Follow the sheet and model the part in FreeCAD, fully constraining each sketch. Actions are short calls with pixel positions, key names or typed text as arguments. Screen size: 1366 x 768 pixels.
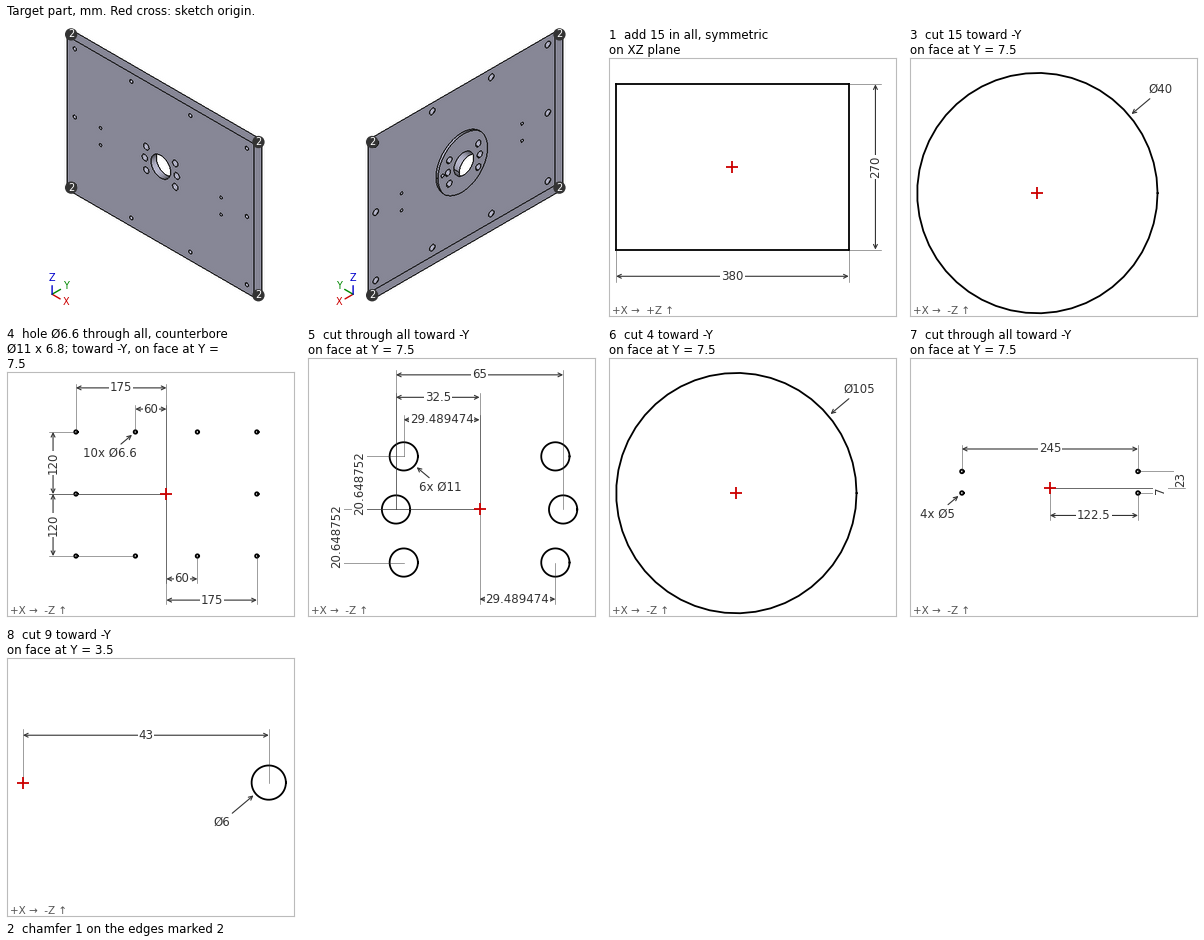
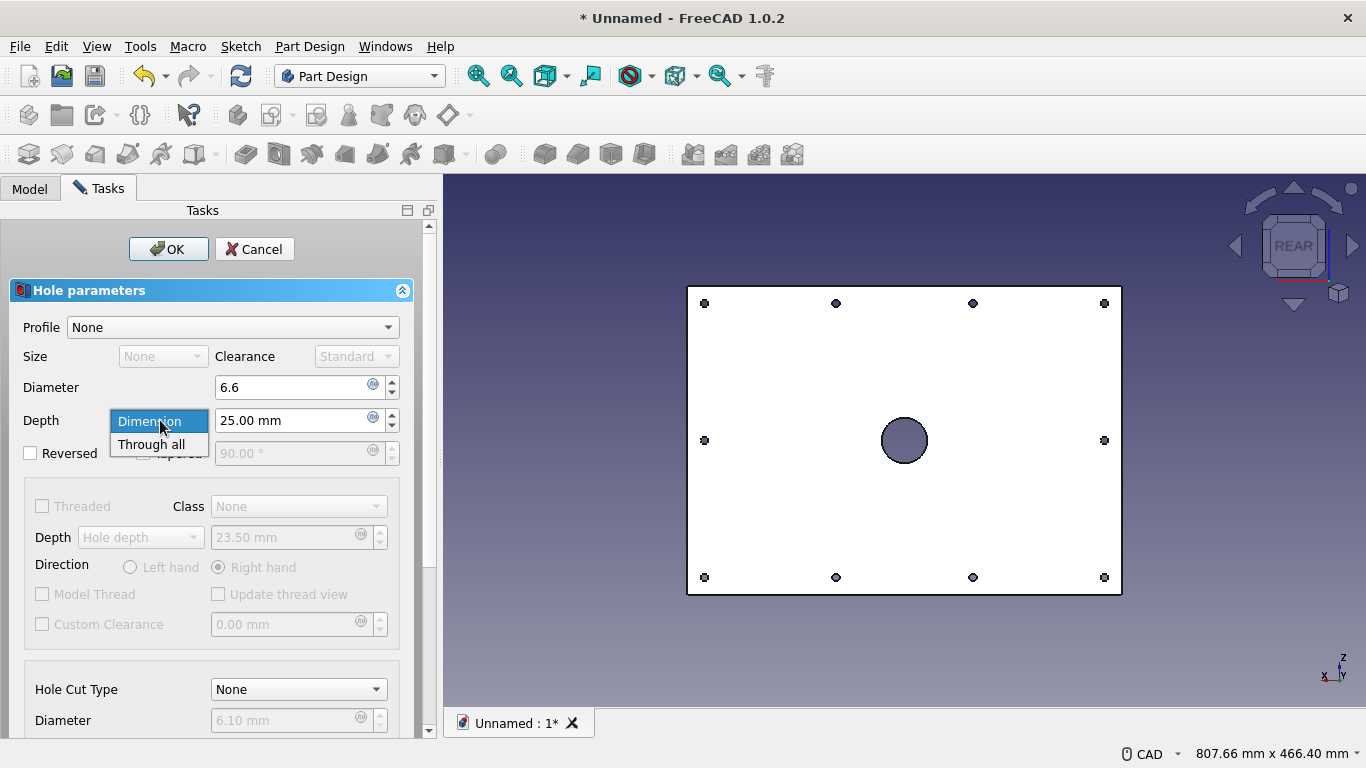
click(158, 444)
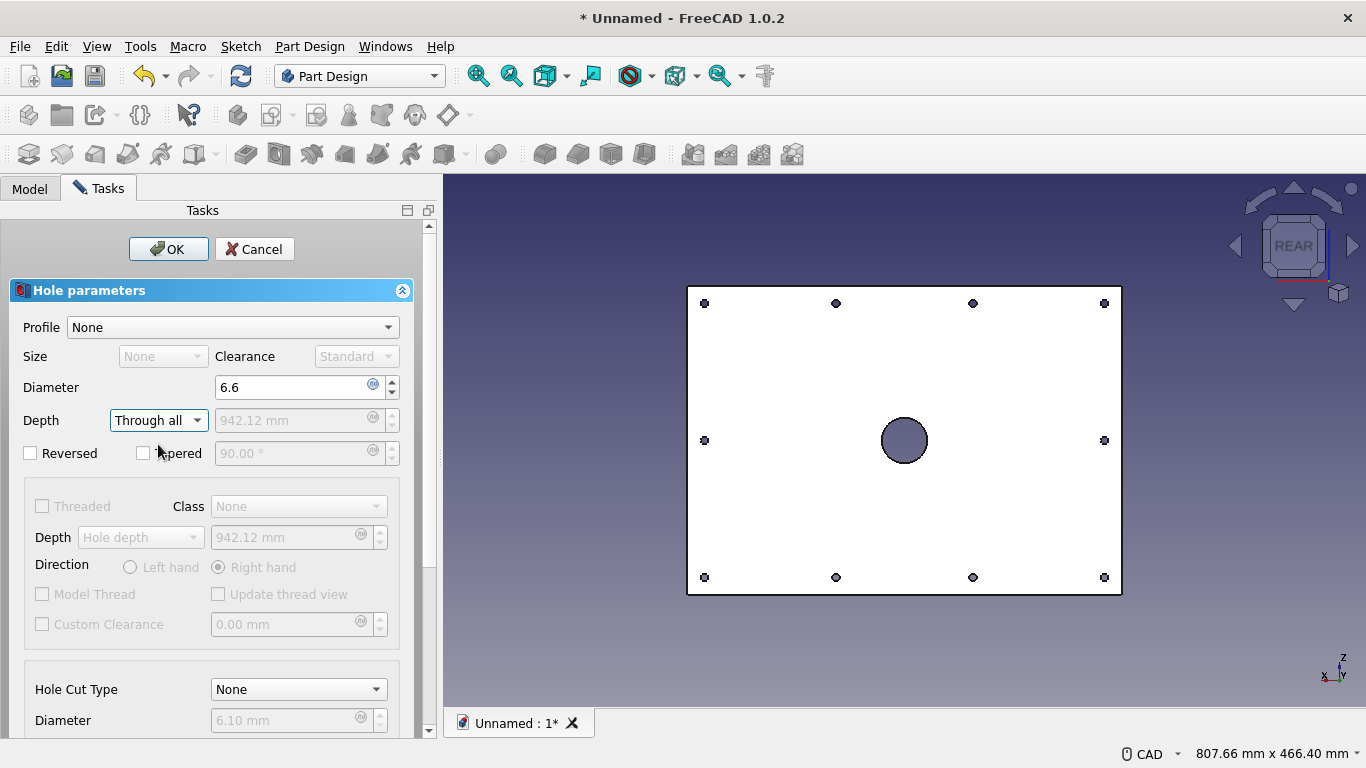
click(300, 690)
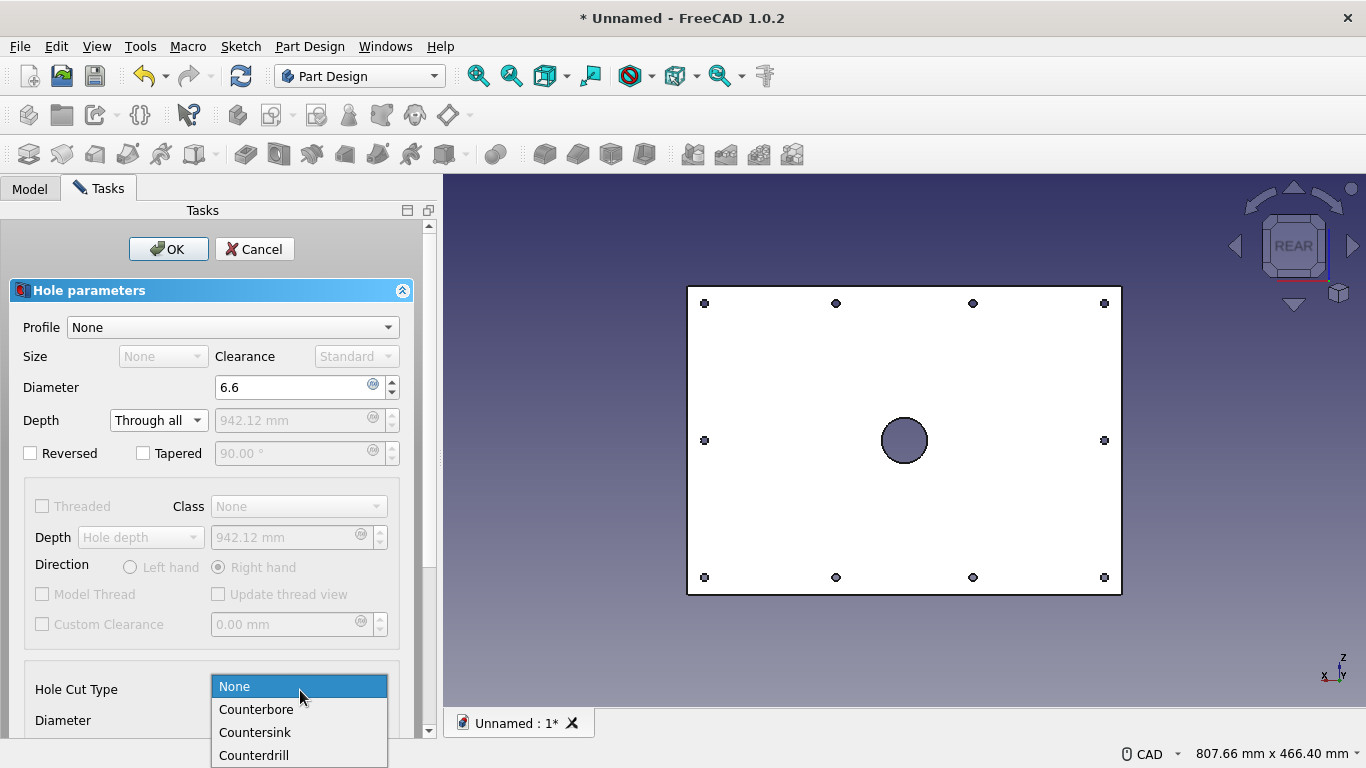
click(298, 710)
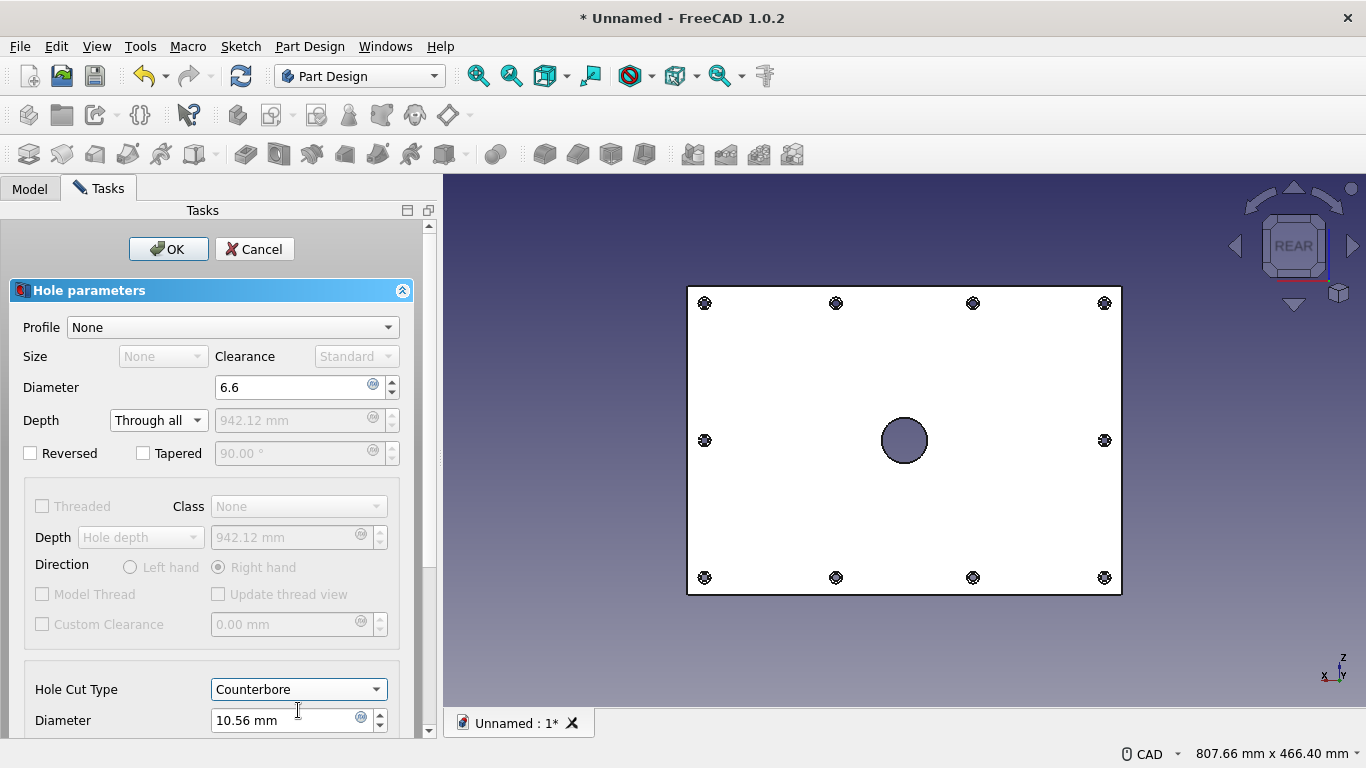
triple_click(292, 720)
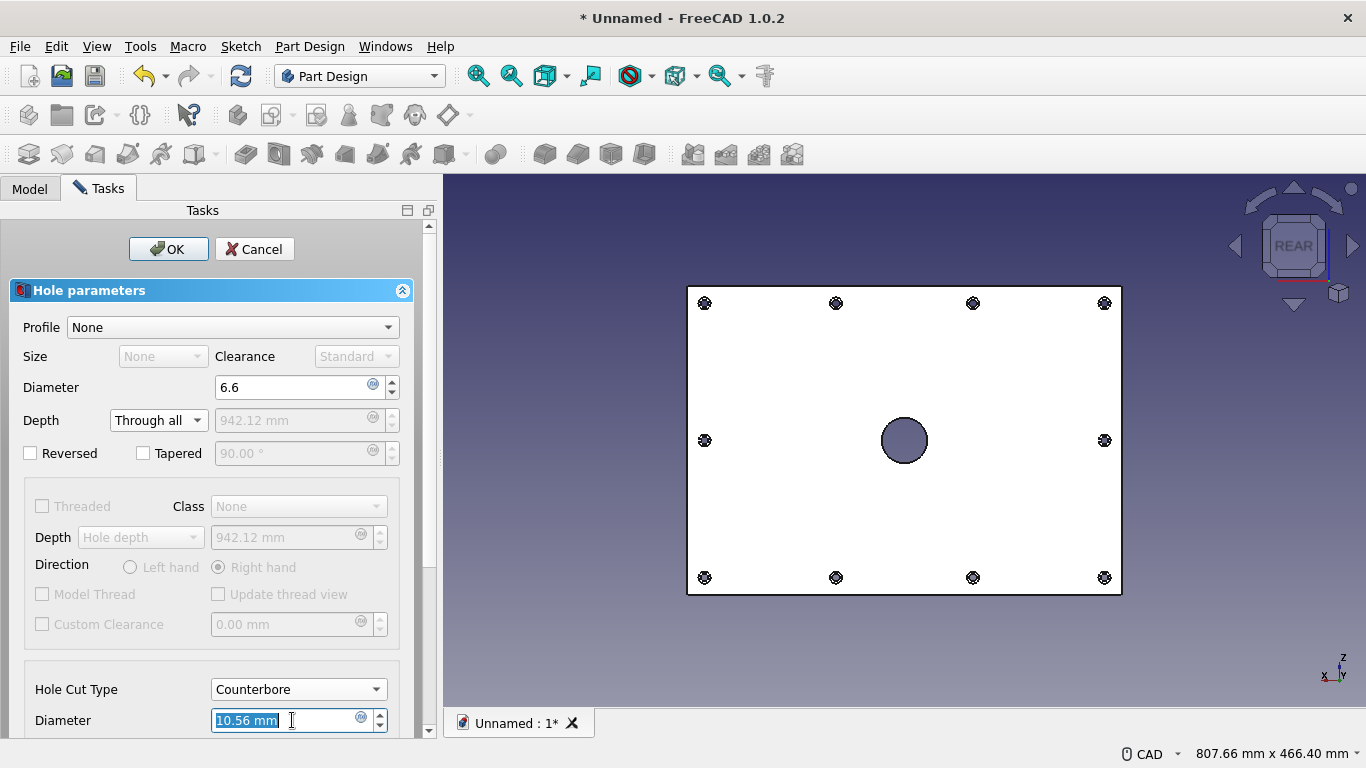
text(11)
key(Tab)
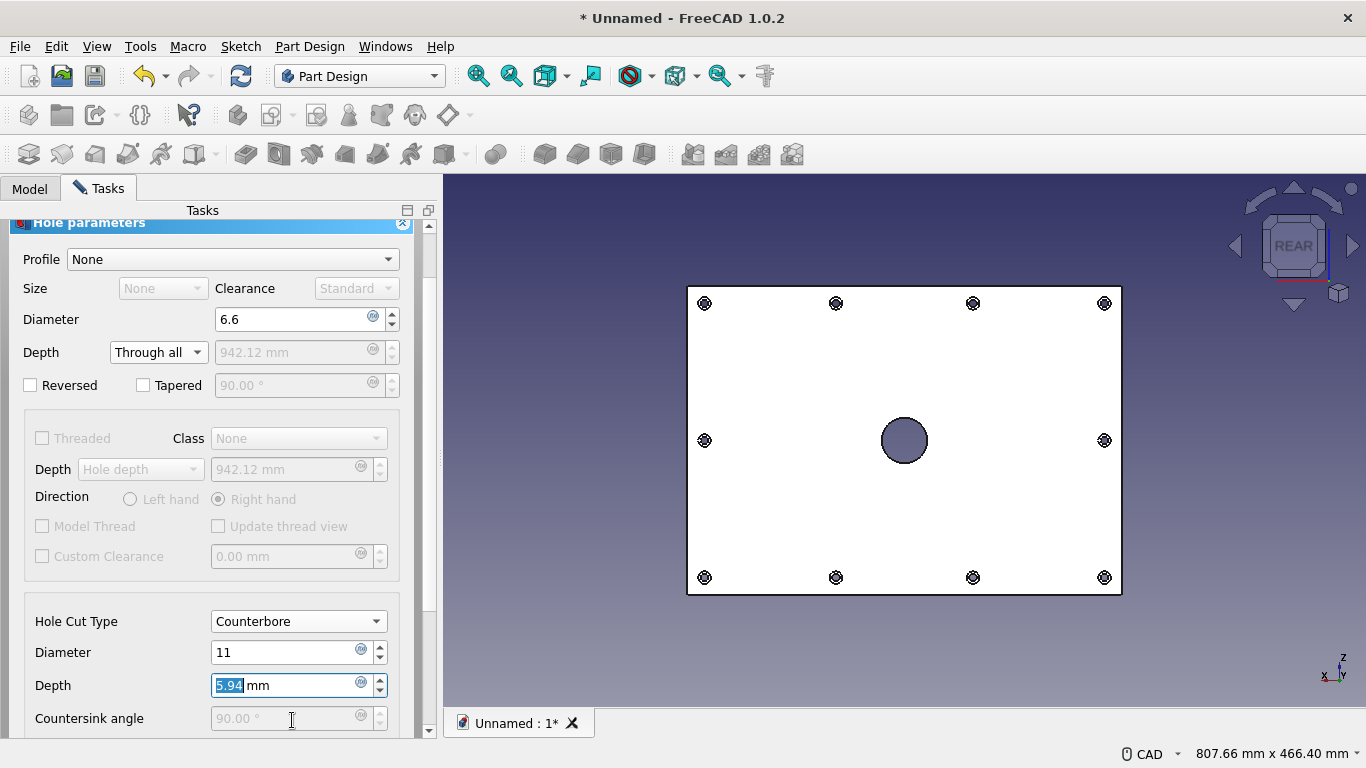
text(6.8)
key(Tab)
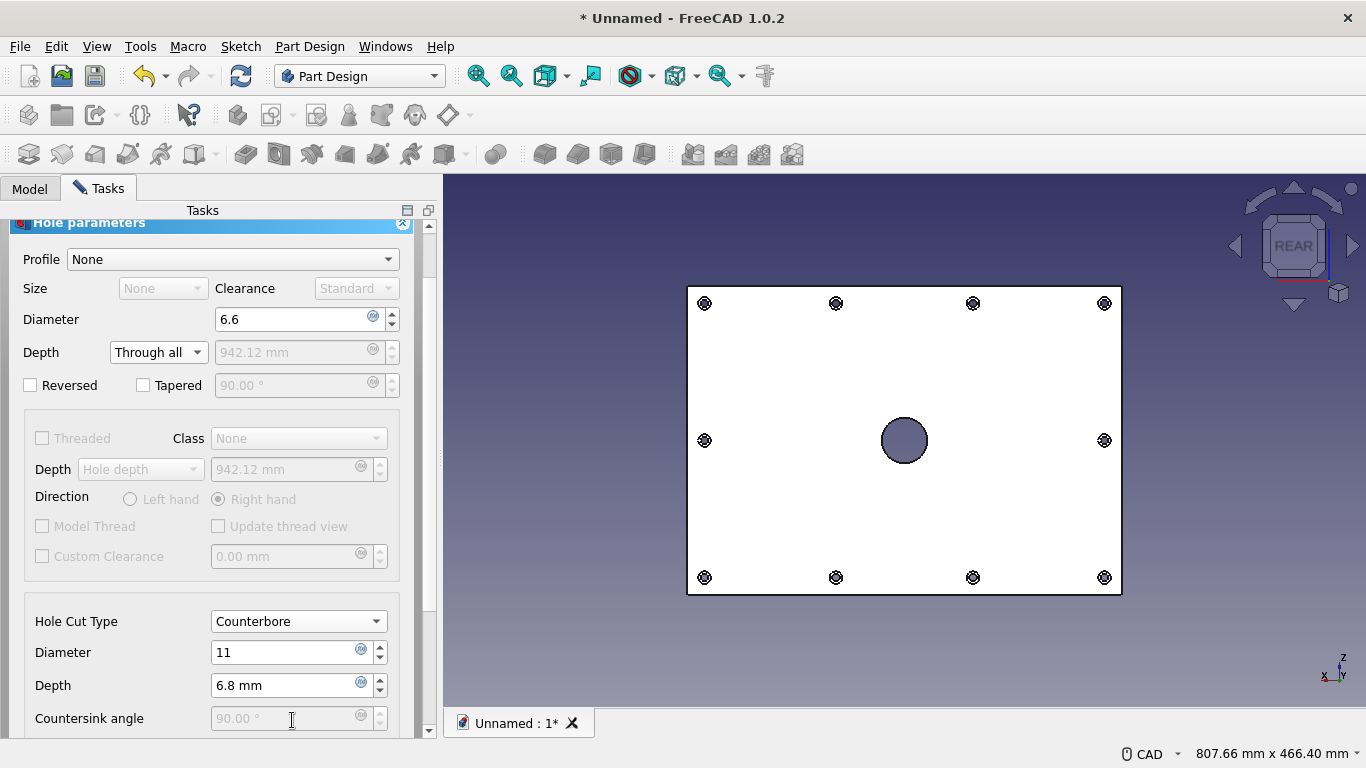
scroll(429, 479, up, 2)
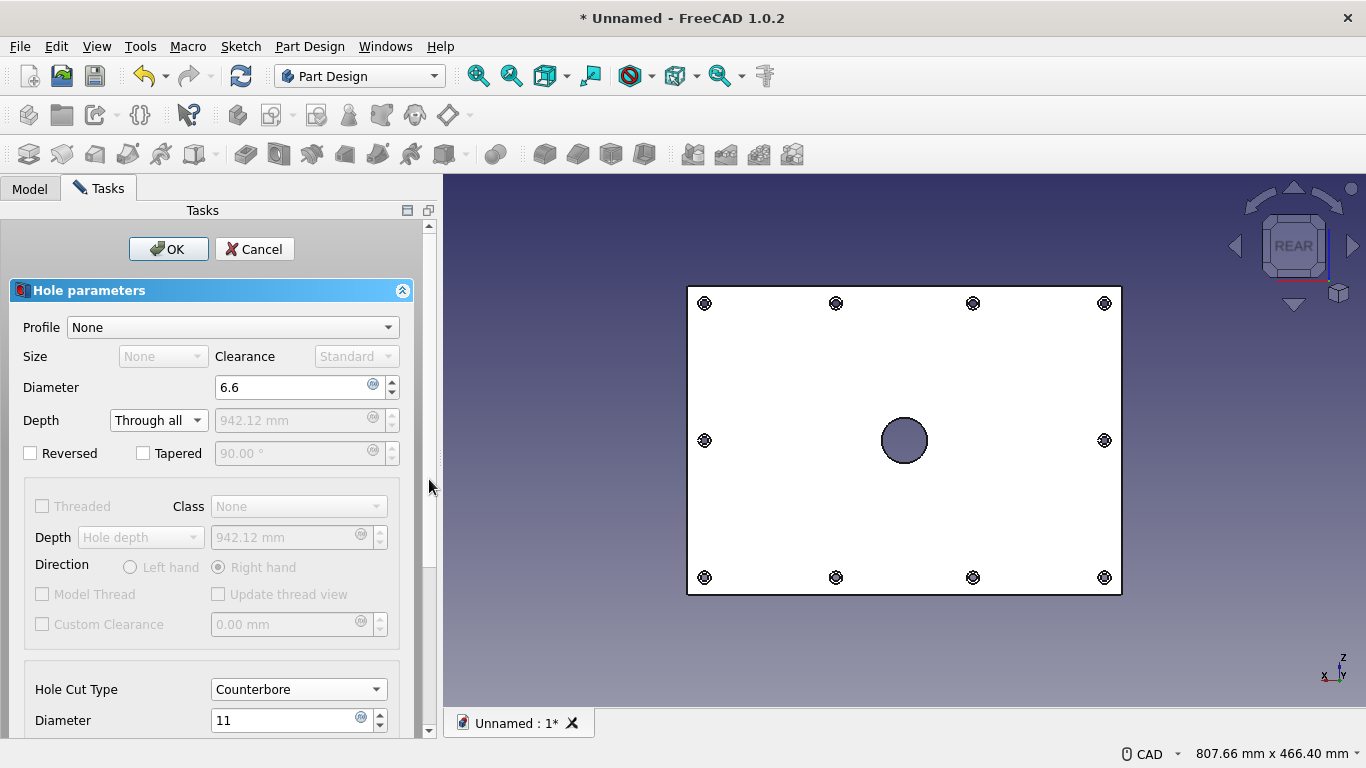
click(169, 249)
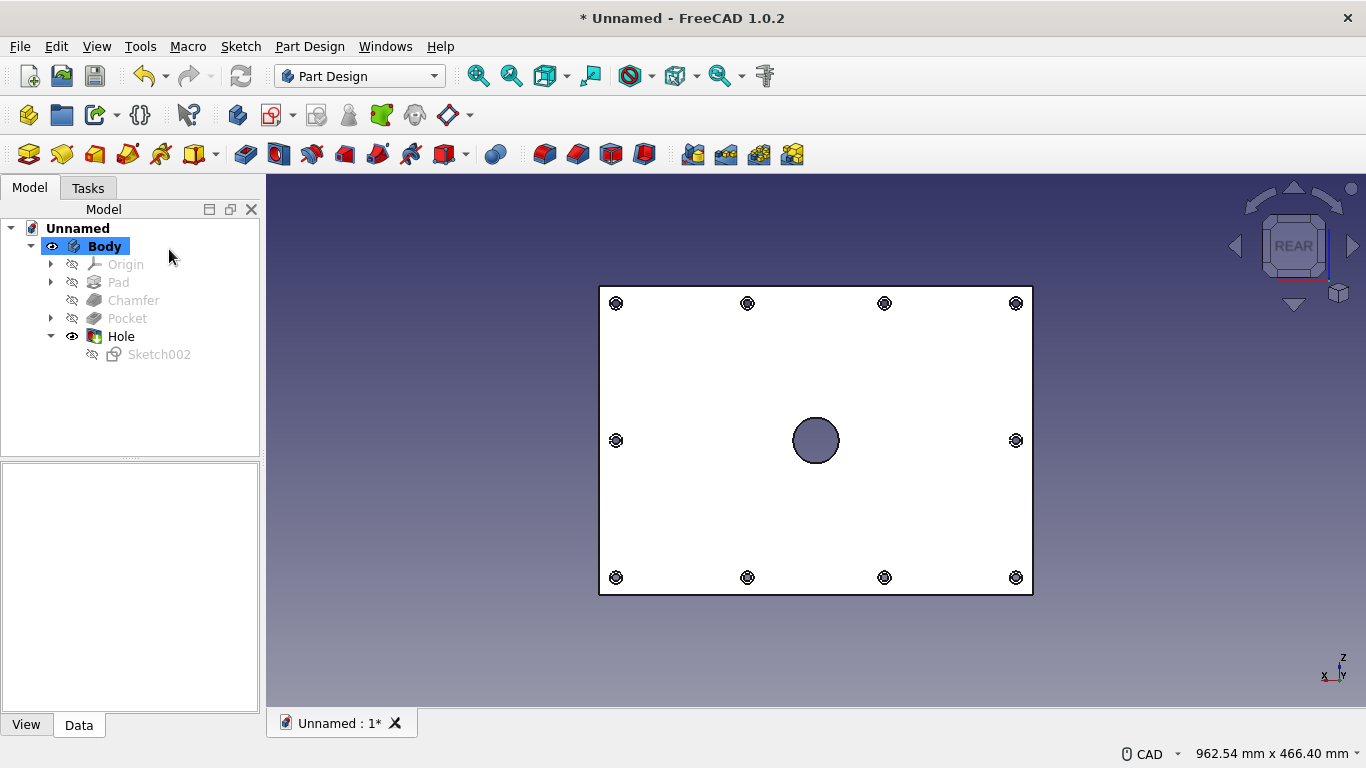
click(692, 395)